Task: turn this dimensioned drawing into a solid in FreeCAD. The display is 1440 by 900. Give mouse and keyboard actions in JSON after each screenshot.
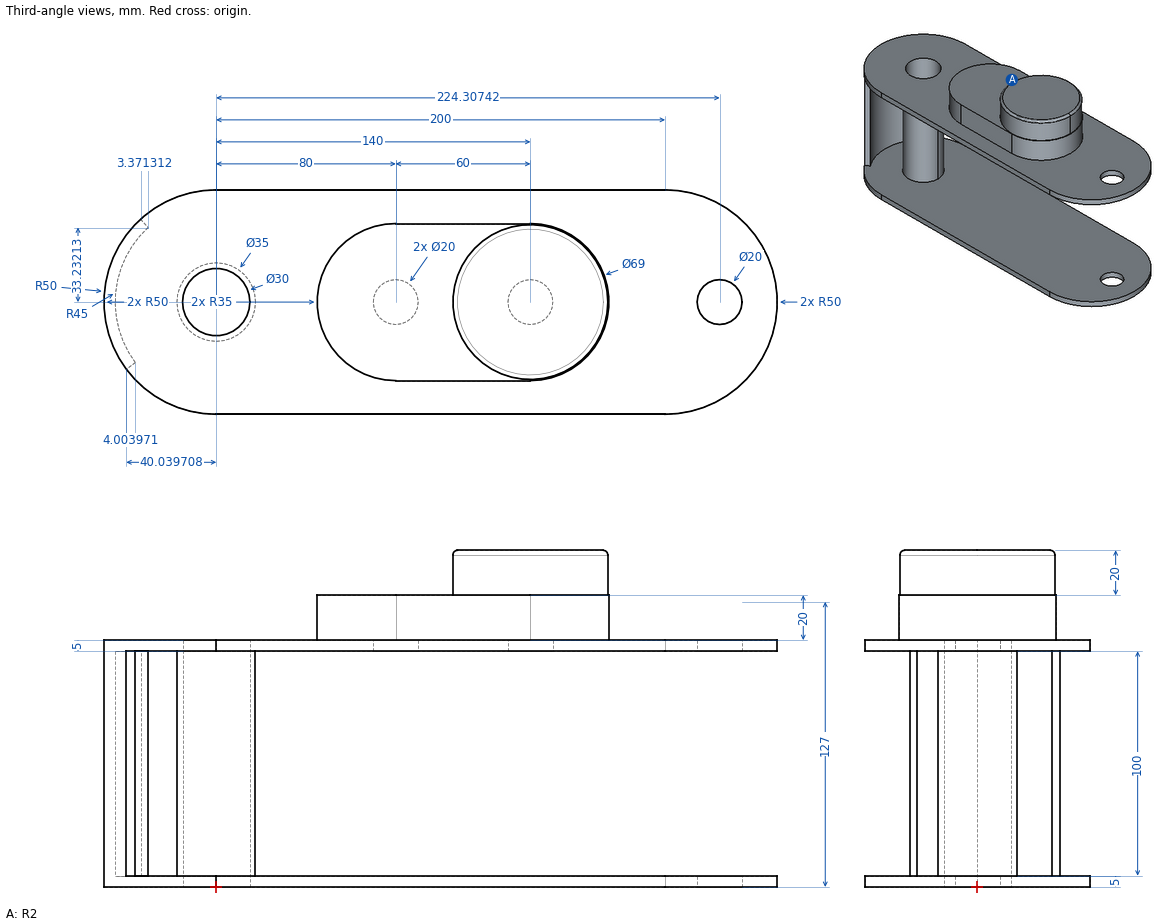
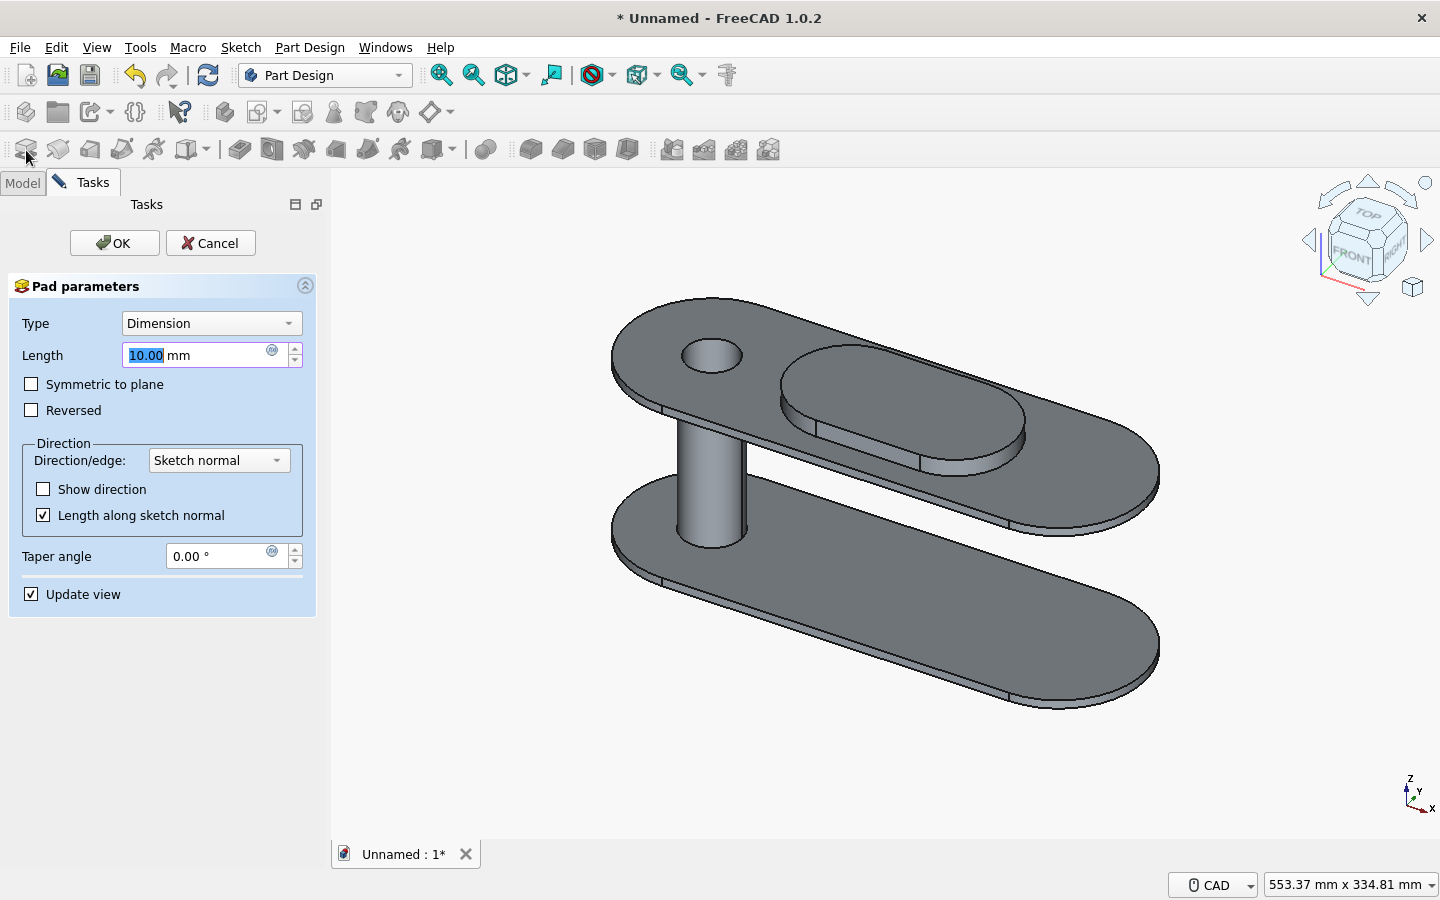
{"action": "type", "text": "20"}
{"action": "key", "text": "Tab"}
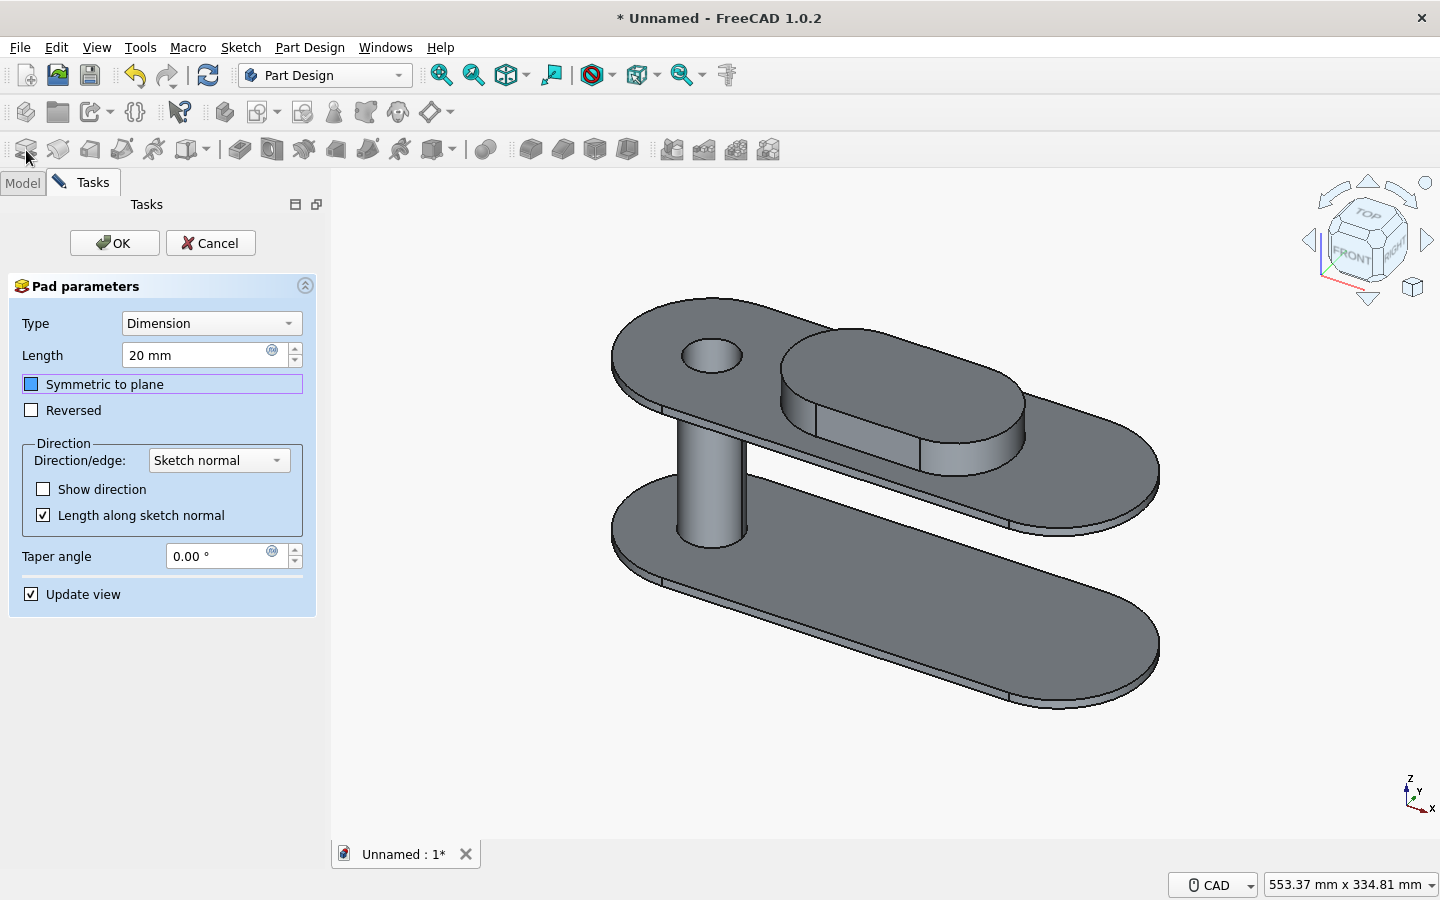
{"action": "left_click", "coordinate": [115, 243]}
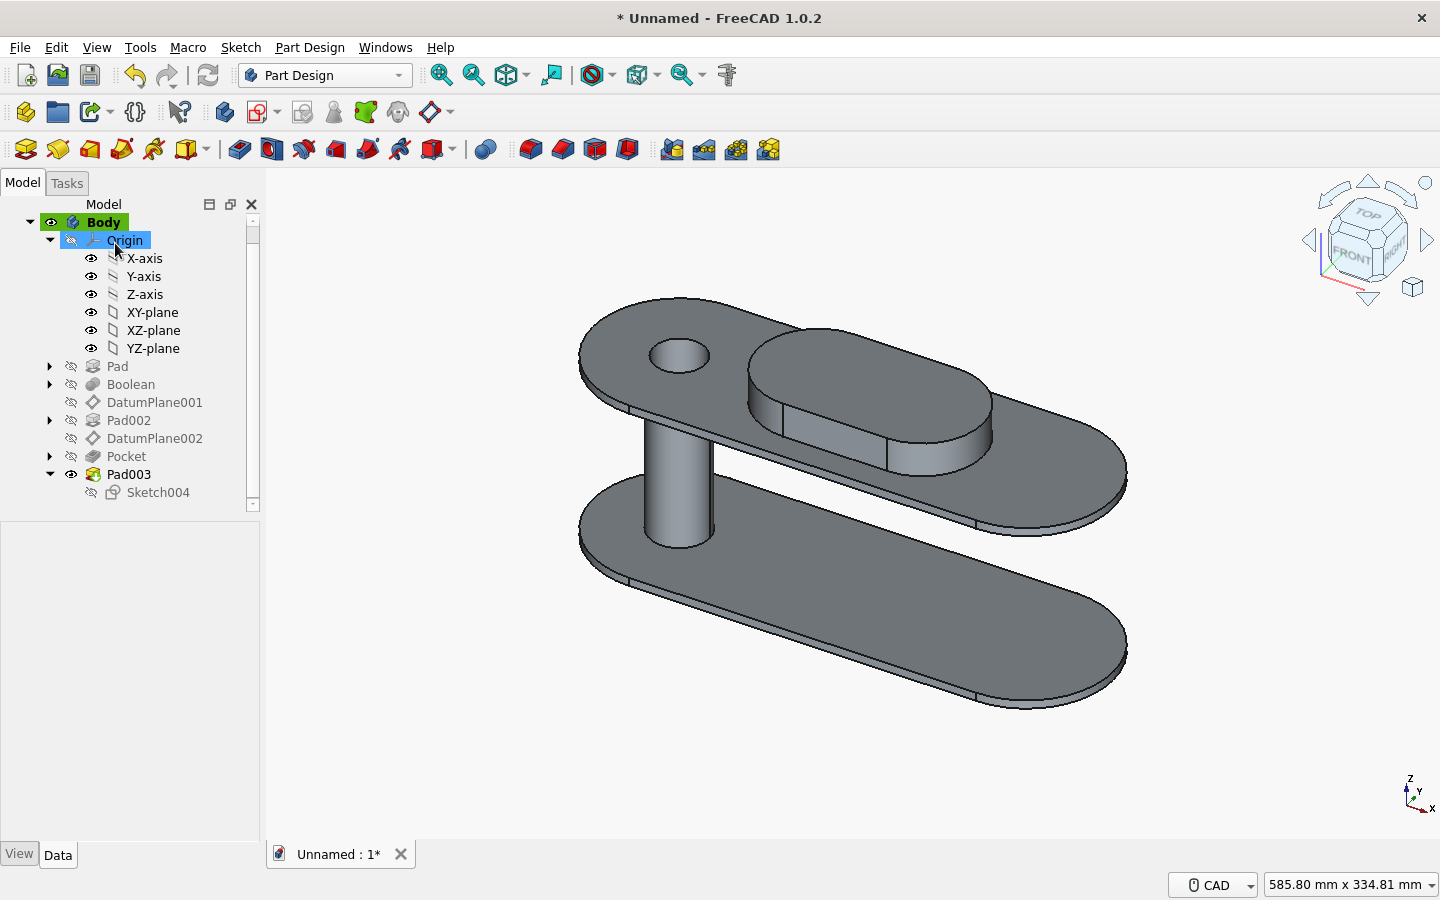
{"action": "left_click", "coordinate": [903, 396]}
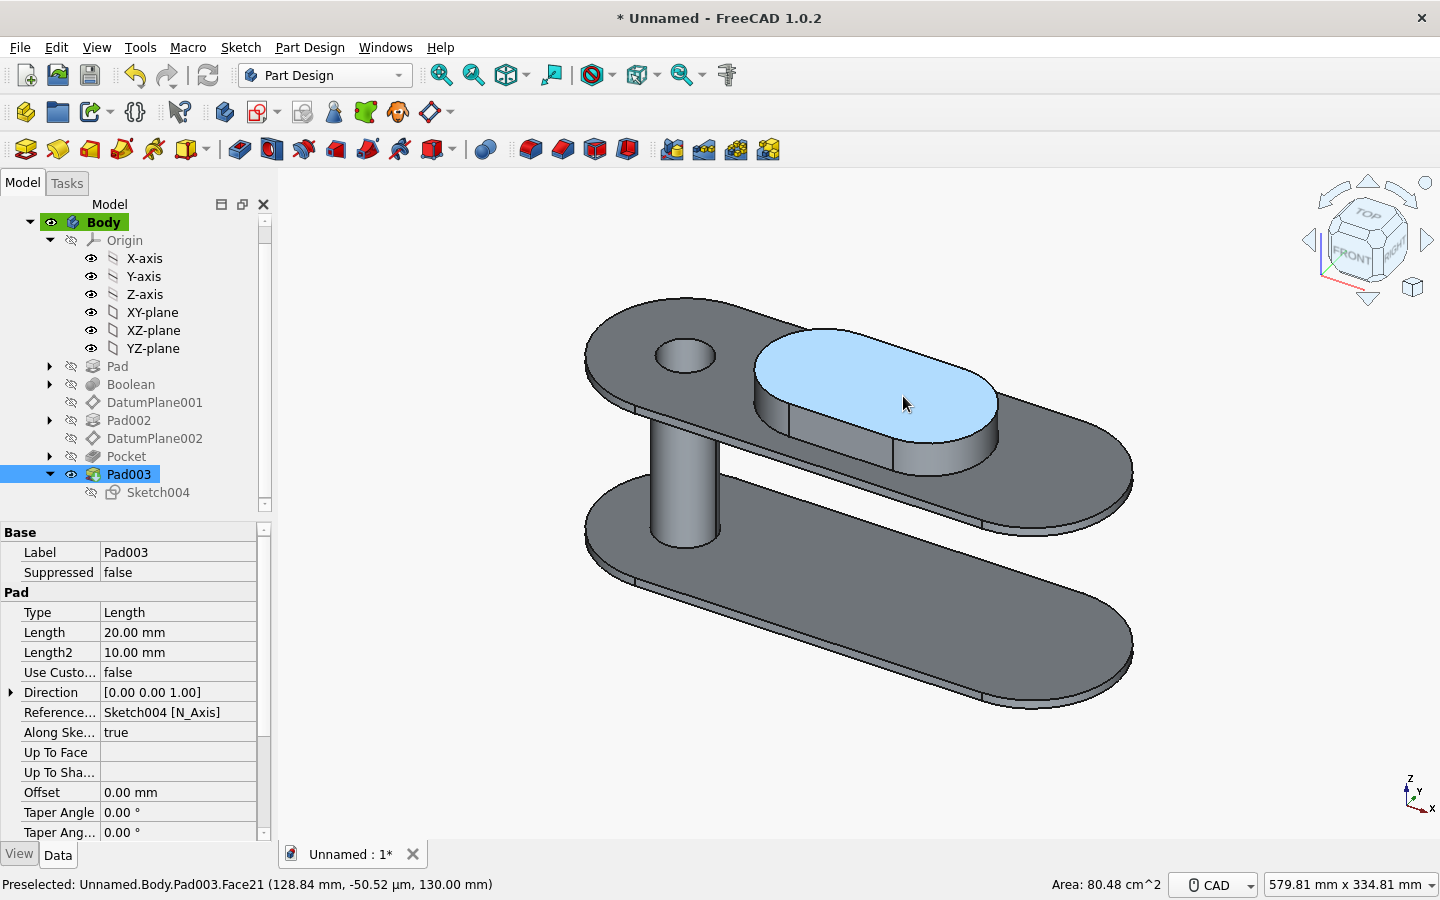
{"action": "left_click", "coordinate": [258, 112]}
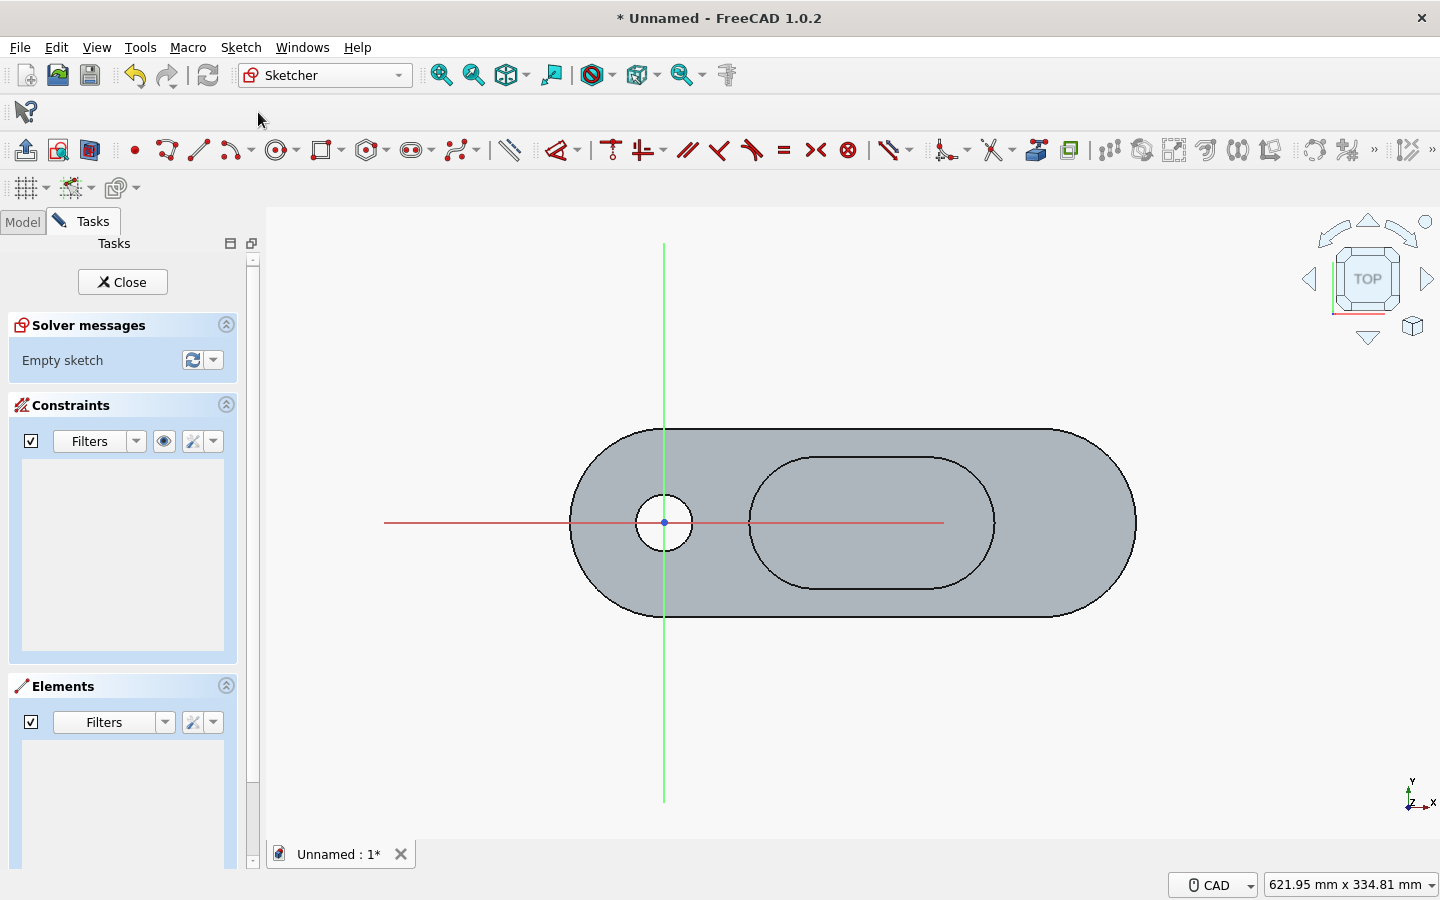
{"action": "scroll", "coordinate": [991, 523], "scroll_direction": "up", "scroll_amount": 6}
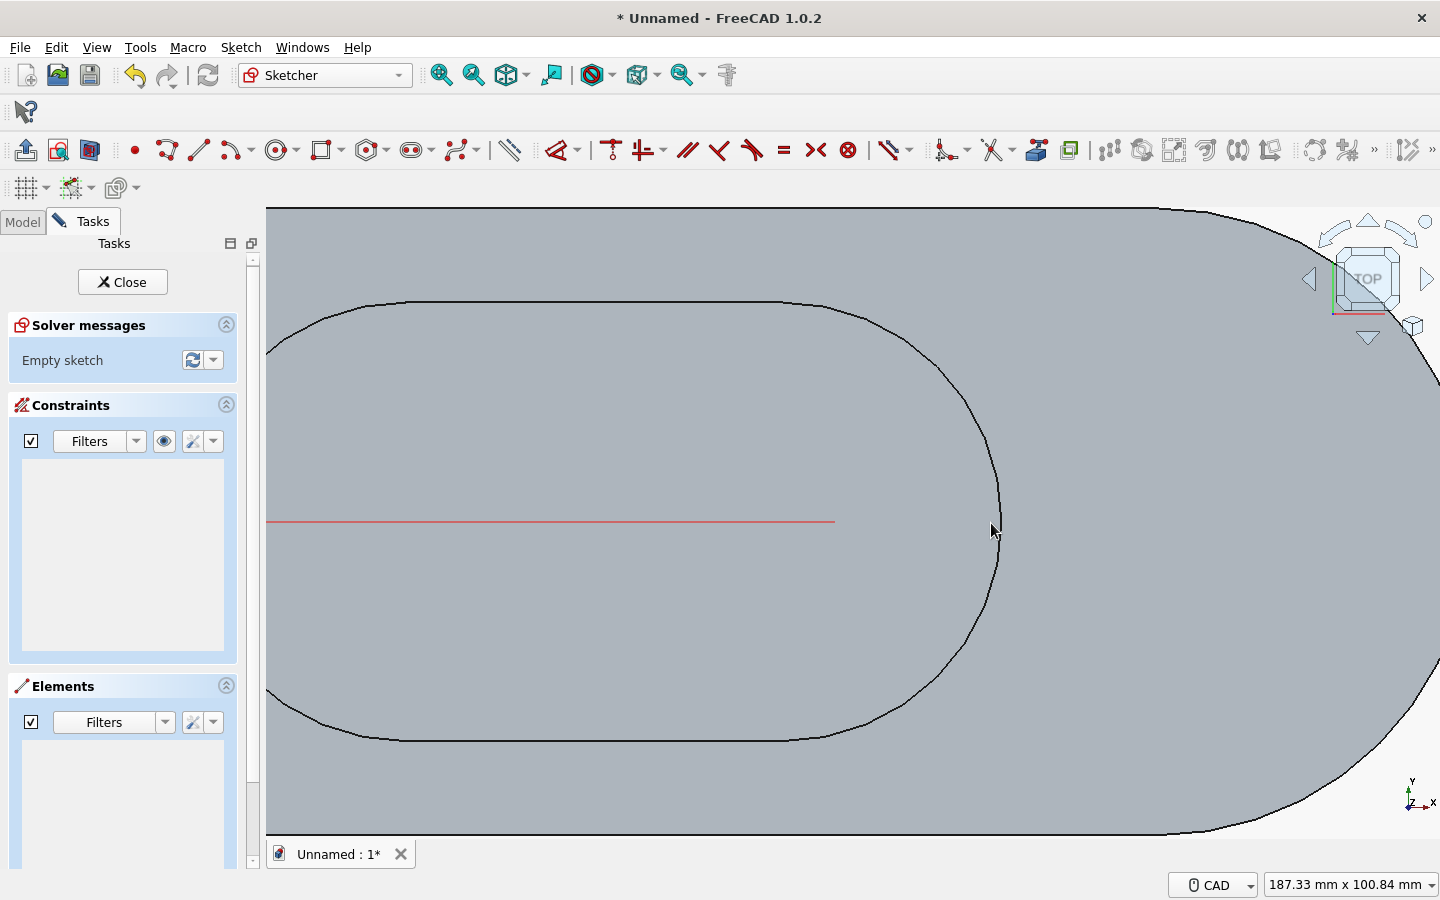
{"action": "left_click", "coordinate": [276, 150]}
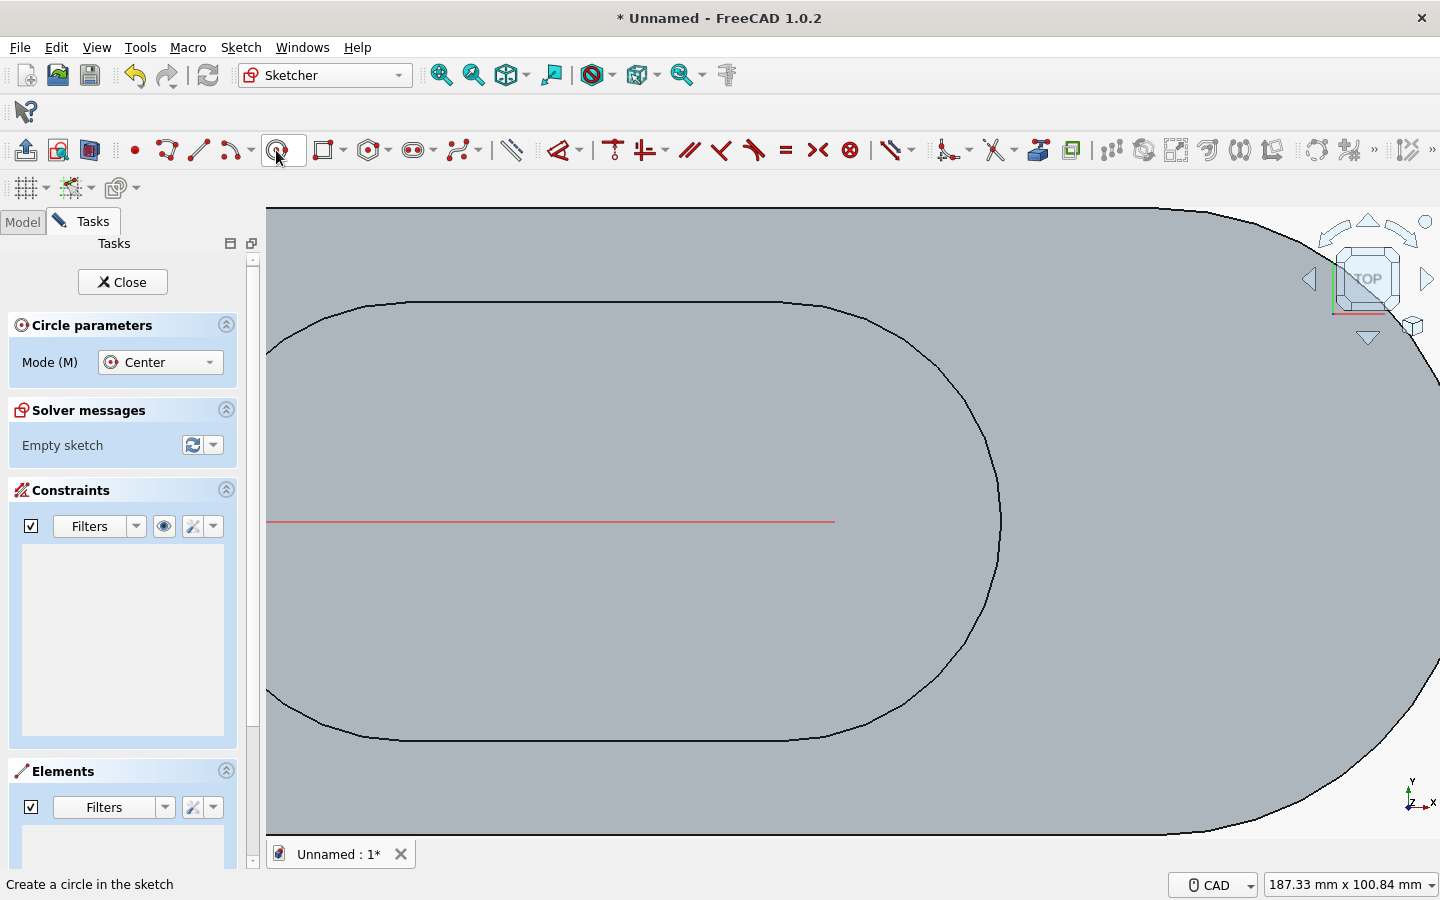
{"action": "left_click", "coordinate": [782, 522]}
{"action": "left_click", "coordinate": [935, 369]}
{"action": "key", "text": "Escape"}